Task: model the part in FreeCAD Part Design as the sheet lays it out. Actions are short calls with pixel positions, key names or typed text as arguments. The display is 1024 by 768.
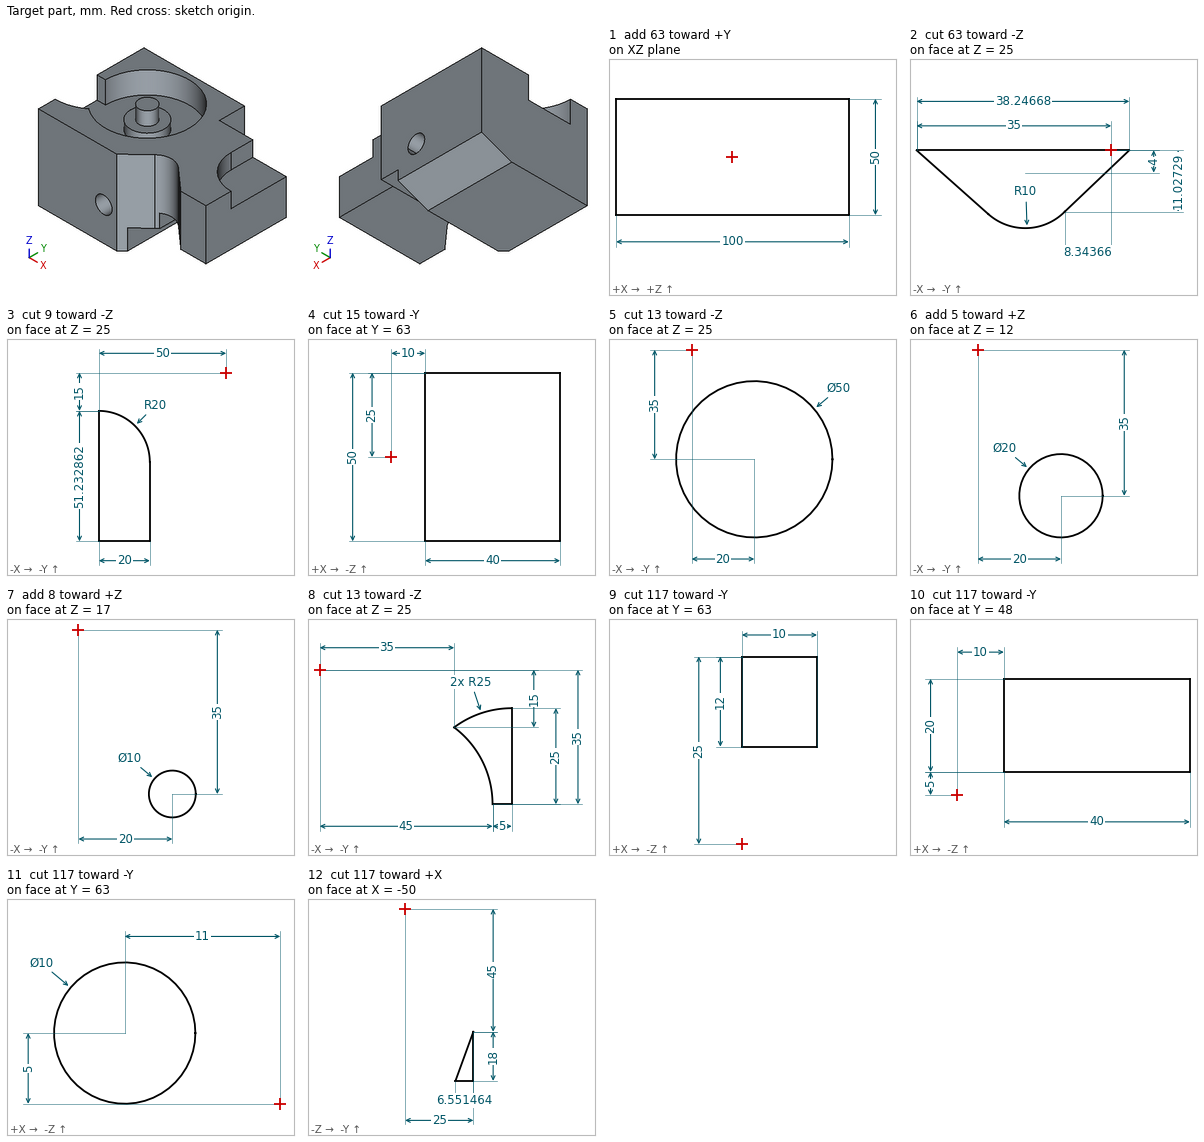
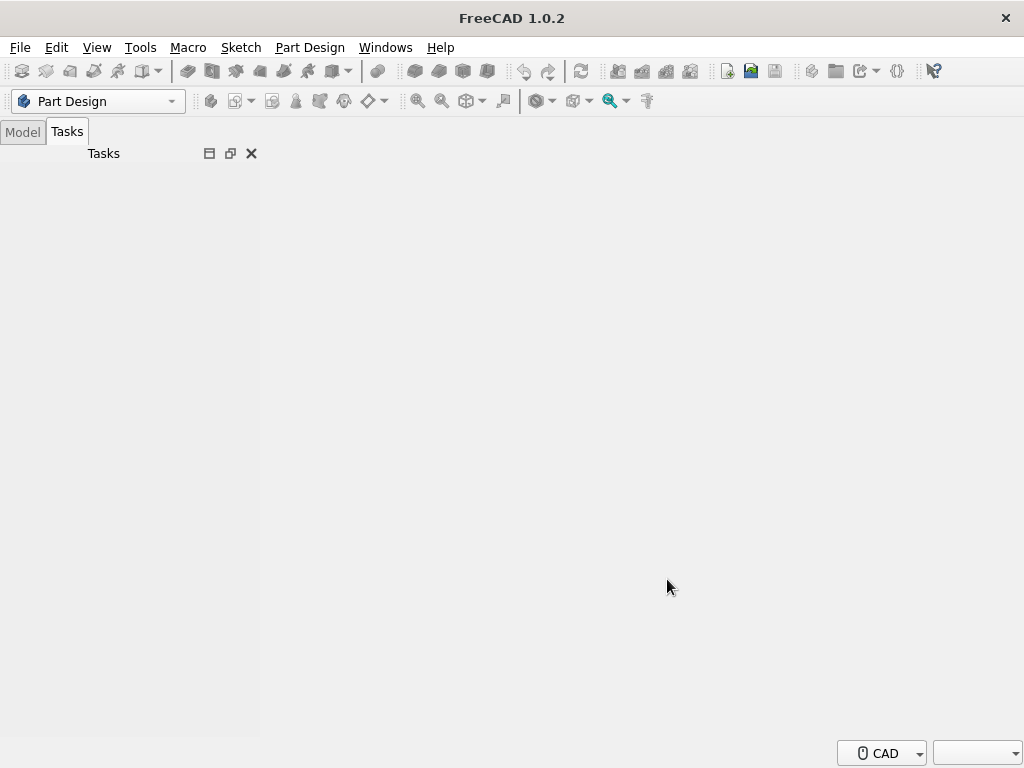
click(728, 72)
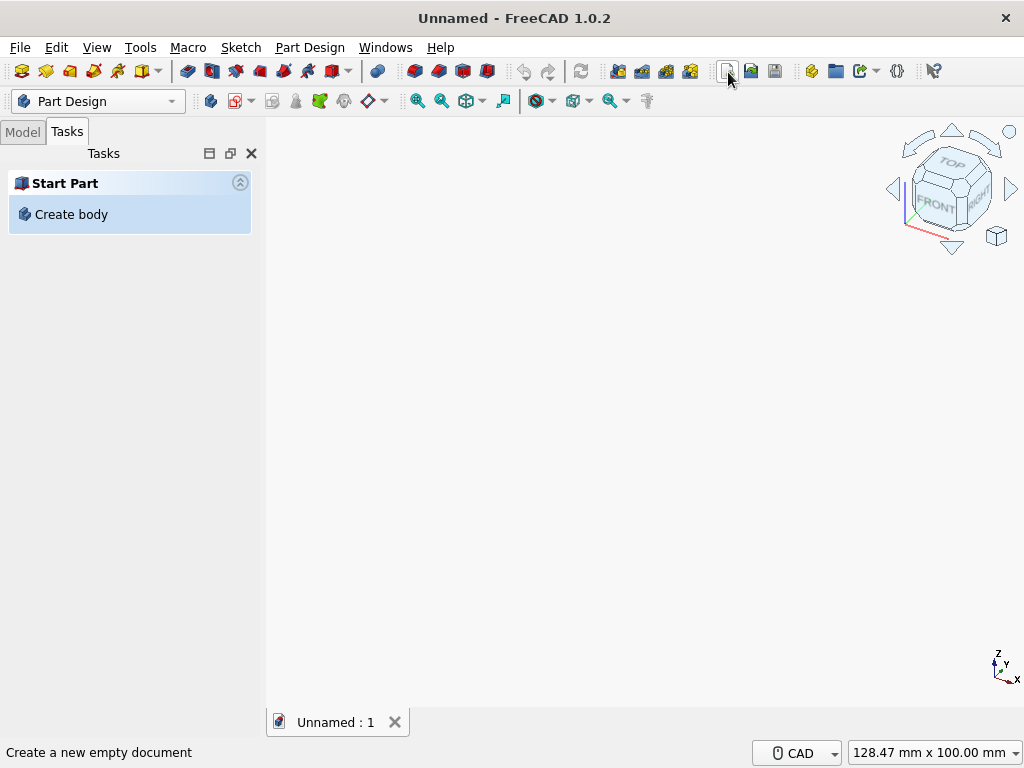
click(236, 102)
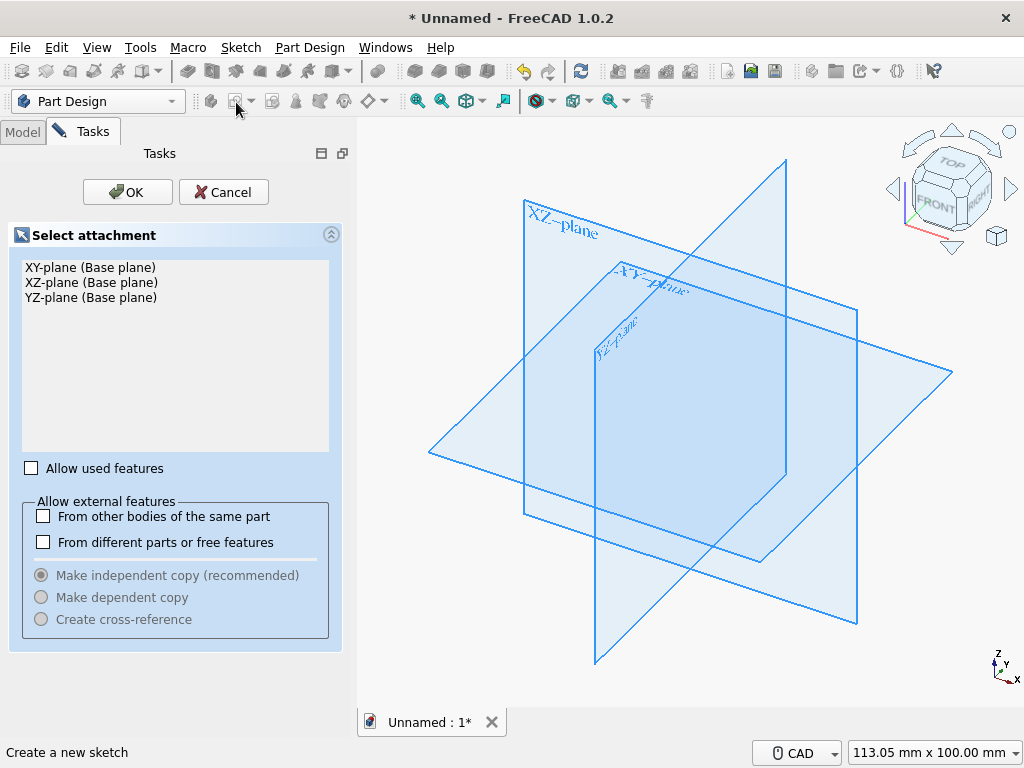
click(82, 282)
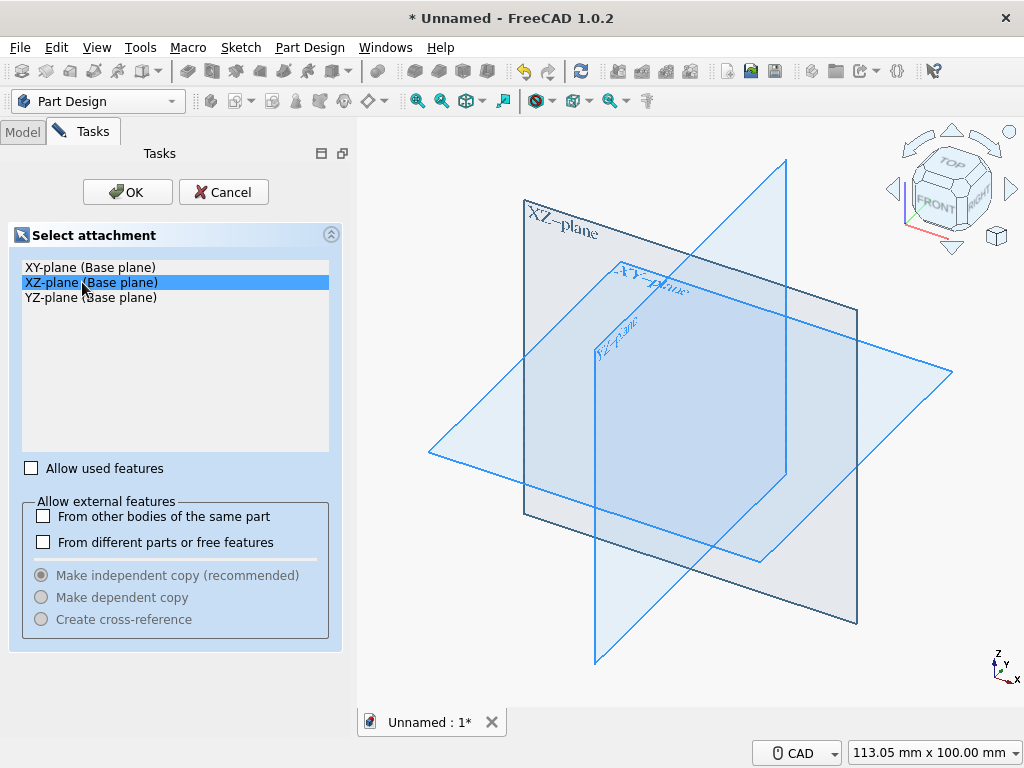
click(128, 192)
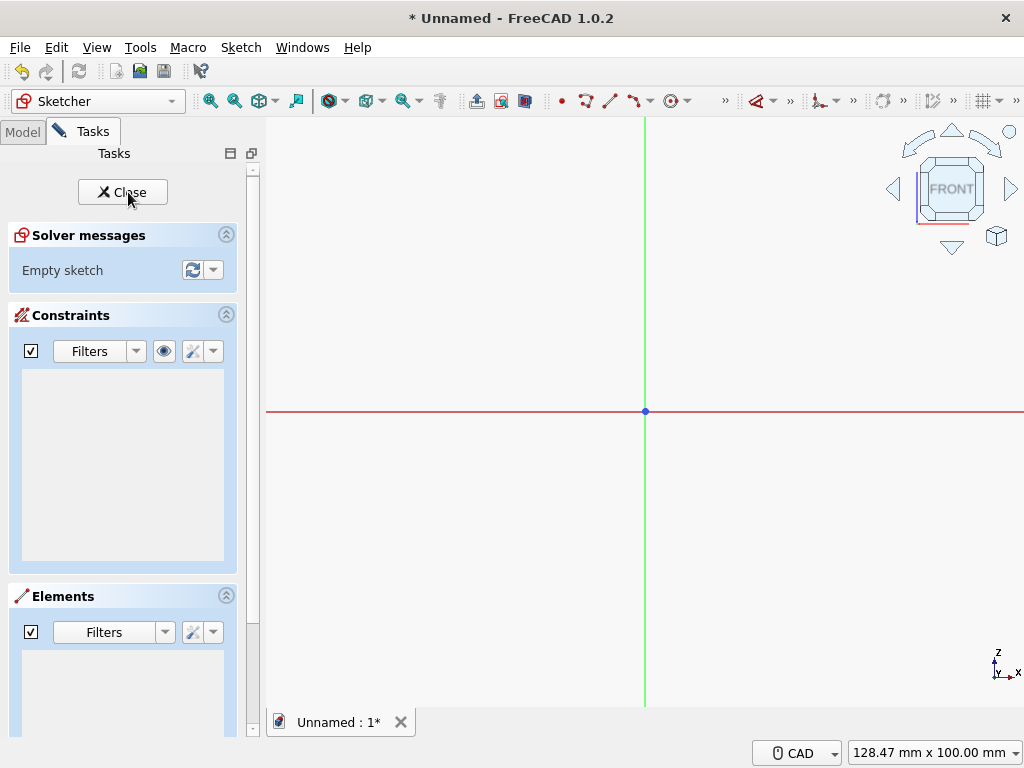
scroll(437, 412, down, 2)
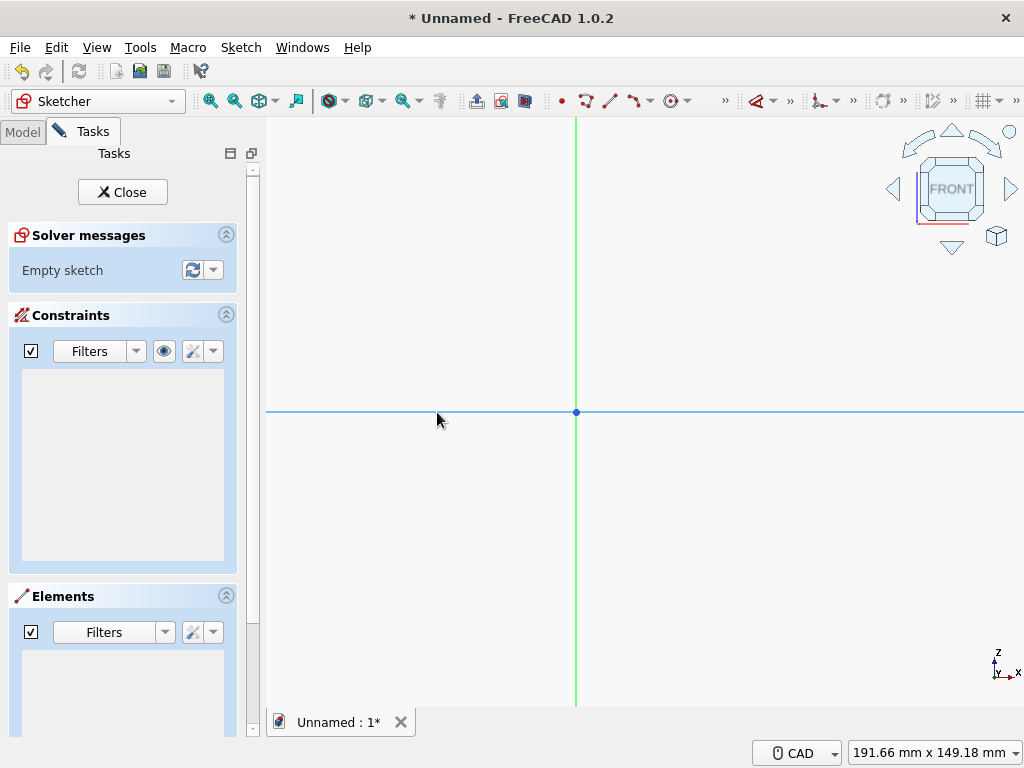
key(g)
key(v)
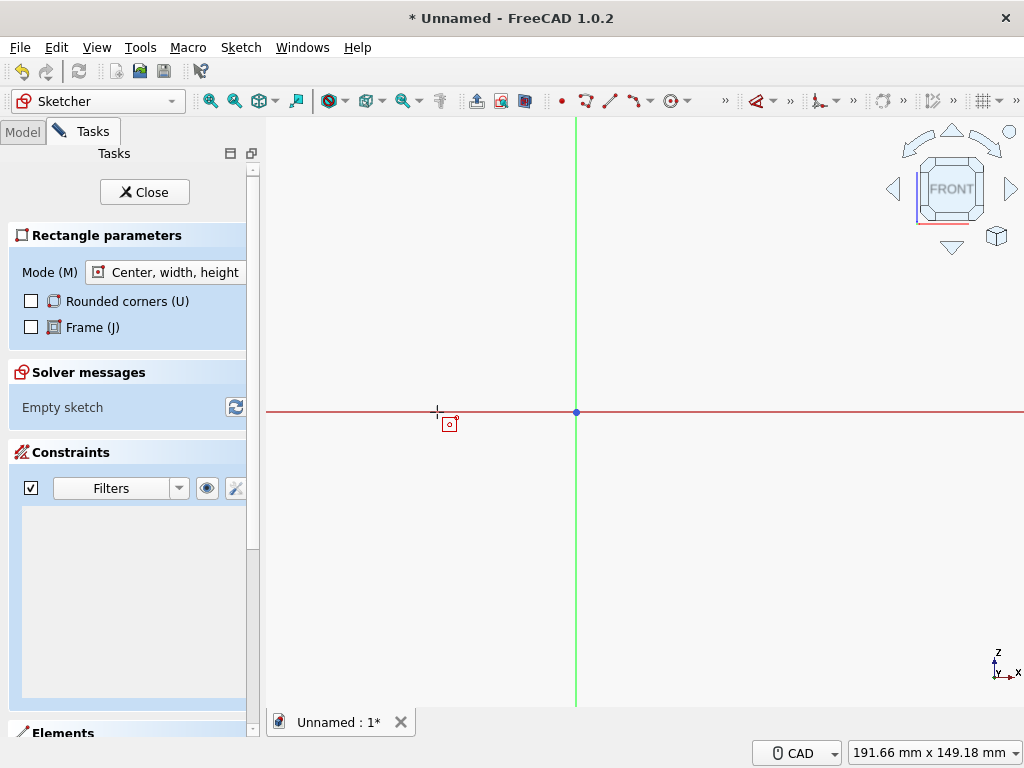
click(577, 412)
click(774, 313)
key(Escape)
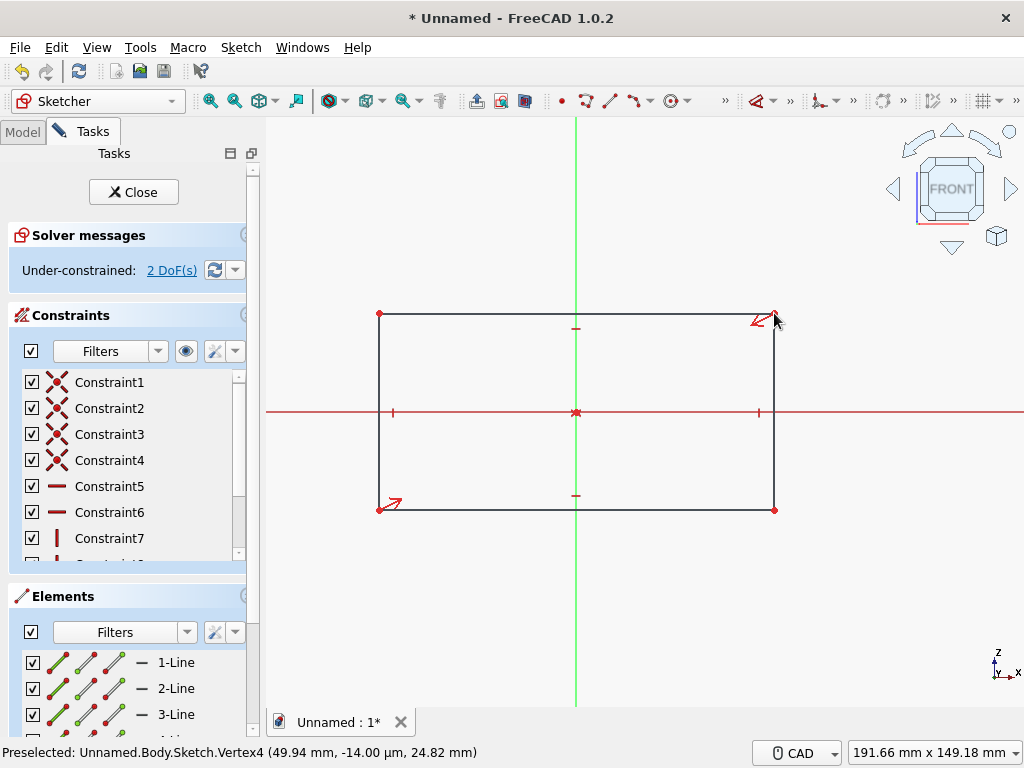
click(774, 451)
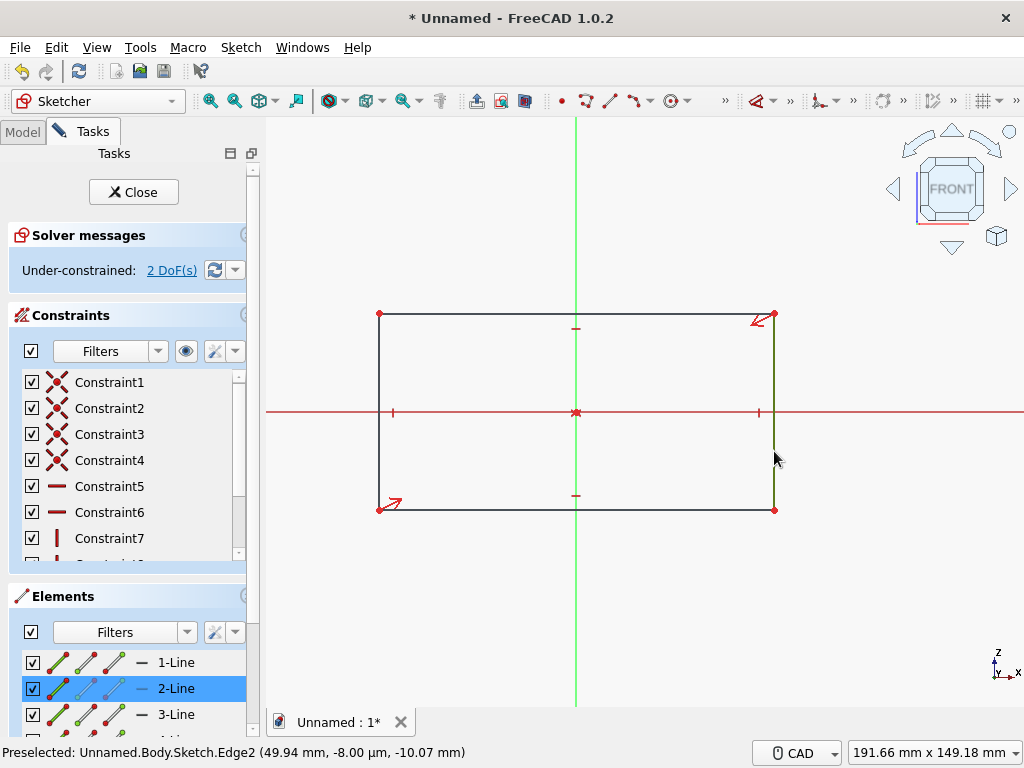
click(776, 102)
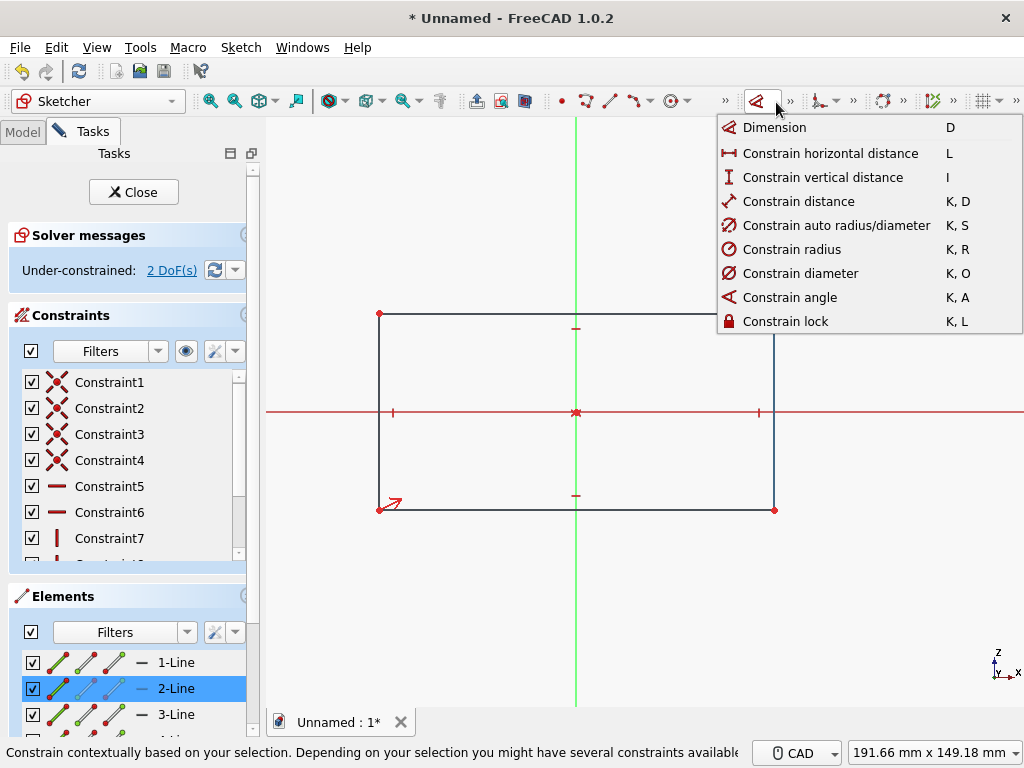
click(870, 177)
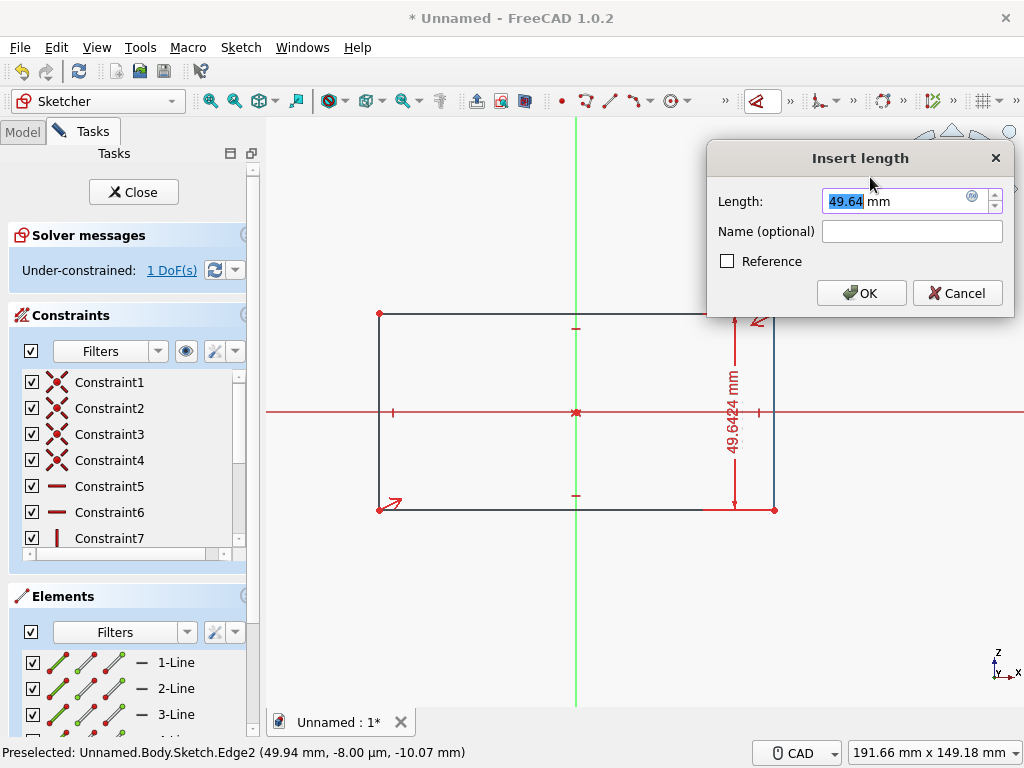
text(50)
key(Return)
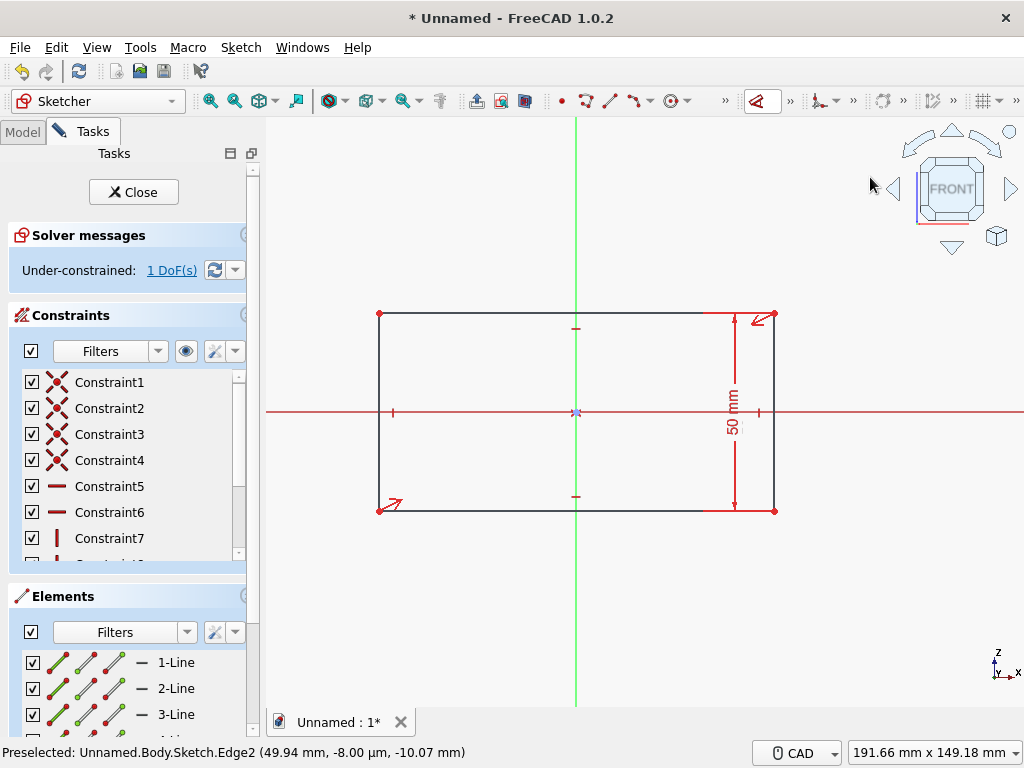
click(498, 511)